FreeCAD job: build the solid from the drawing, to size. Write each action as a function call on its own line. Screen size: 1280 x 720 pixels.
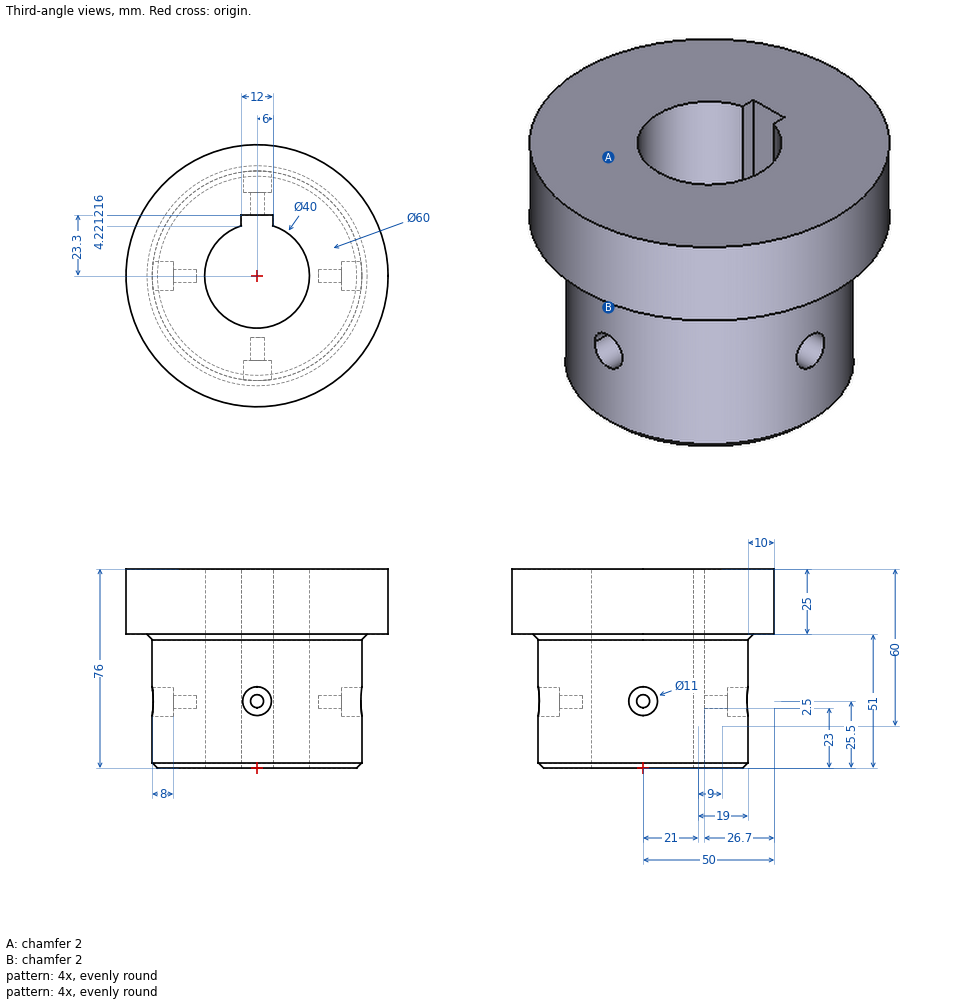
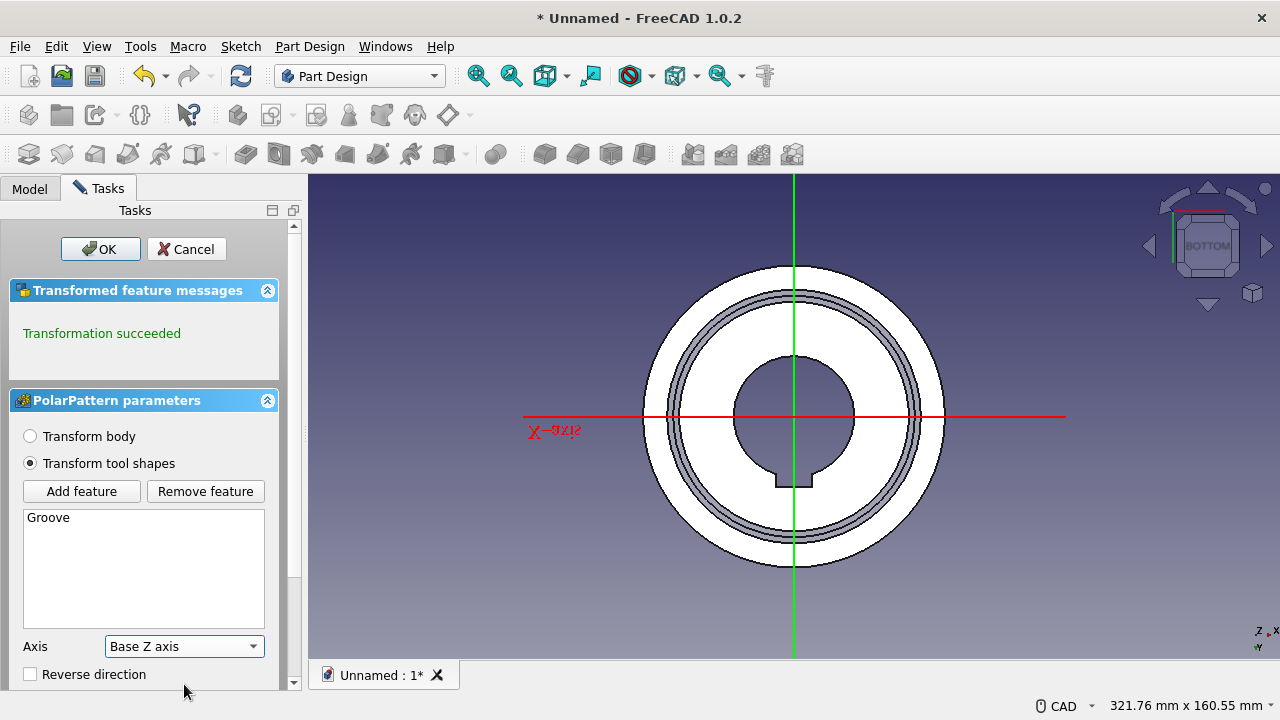
scroll(294, 455, down, 3)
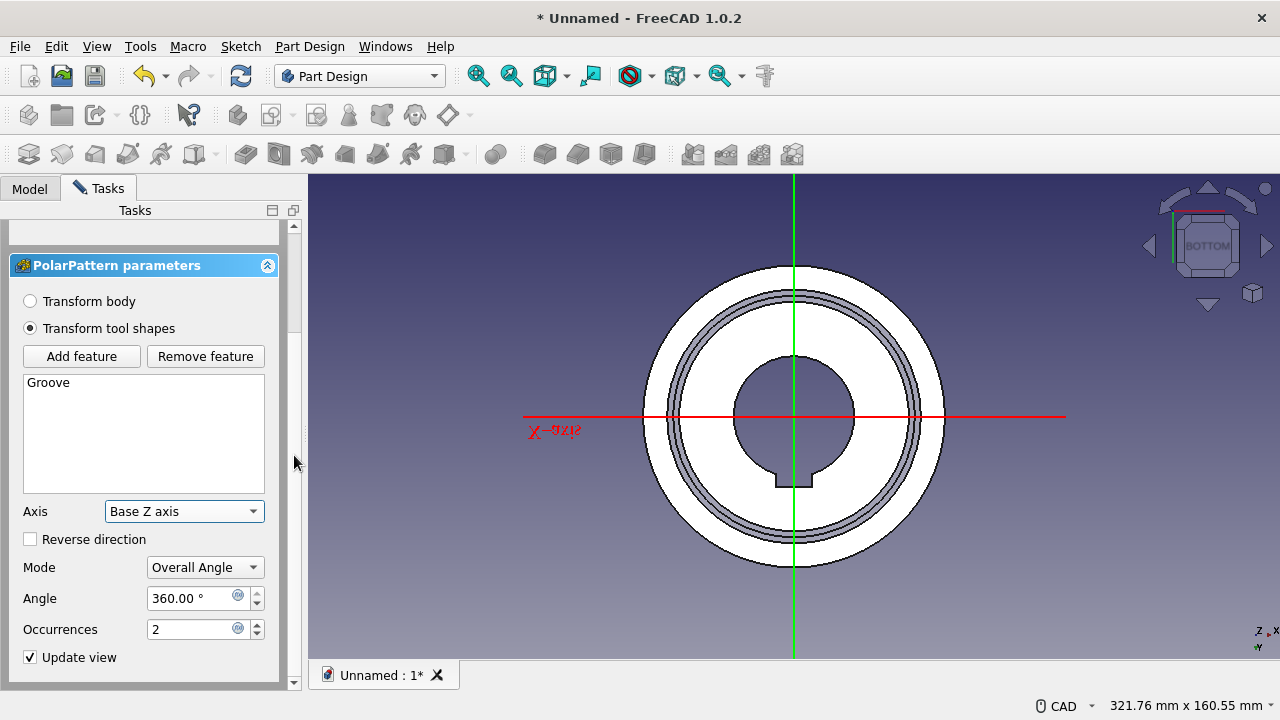
triple_click(199, 630)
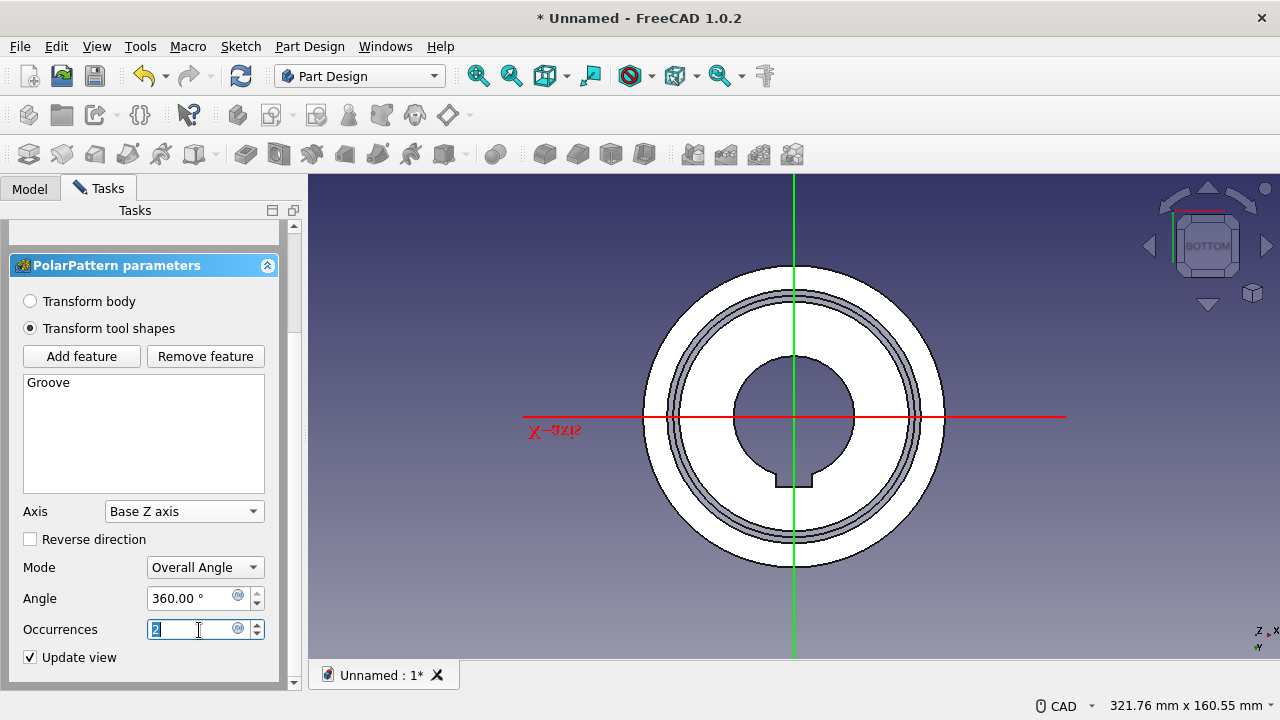
text(4)
key(Tab)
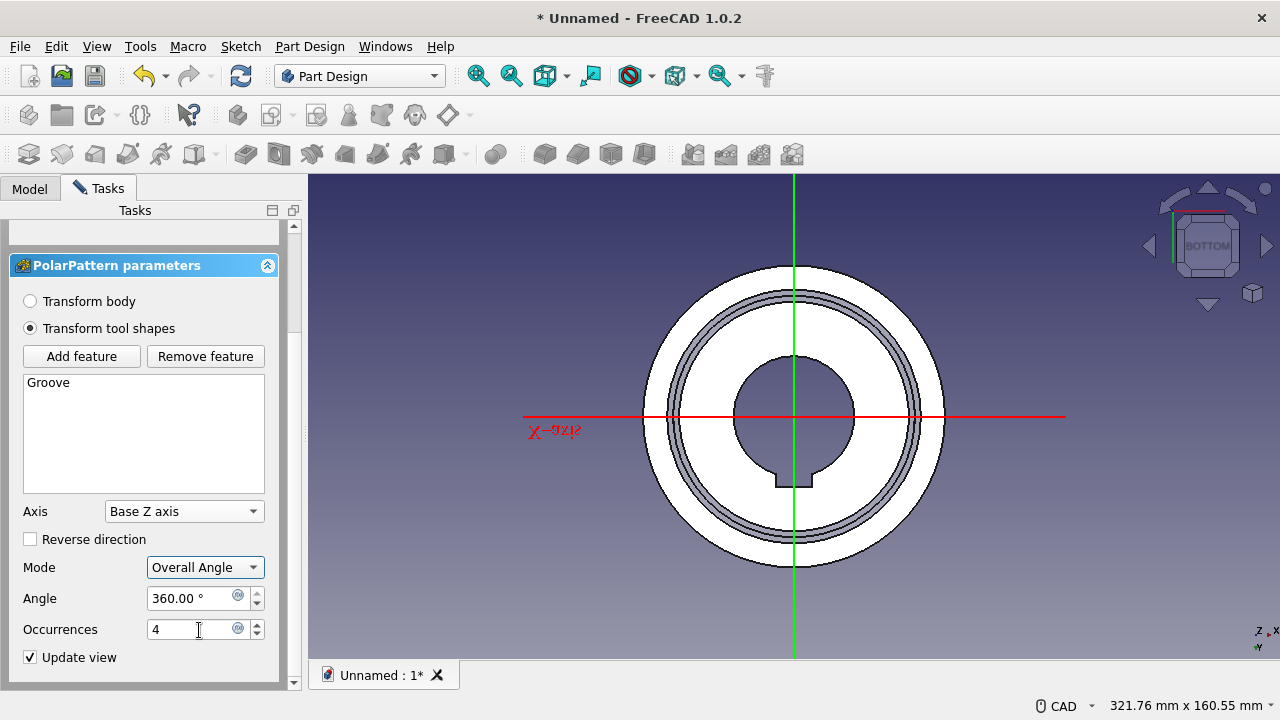
scroll(294, 455, up, 3)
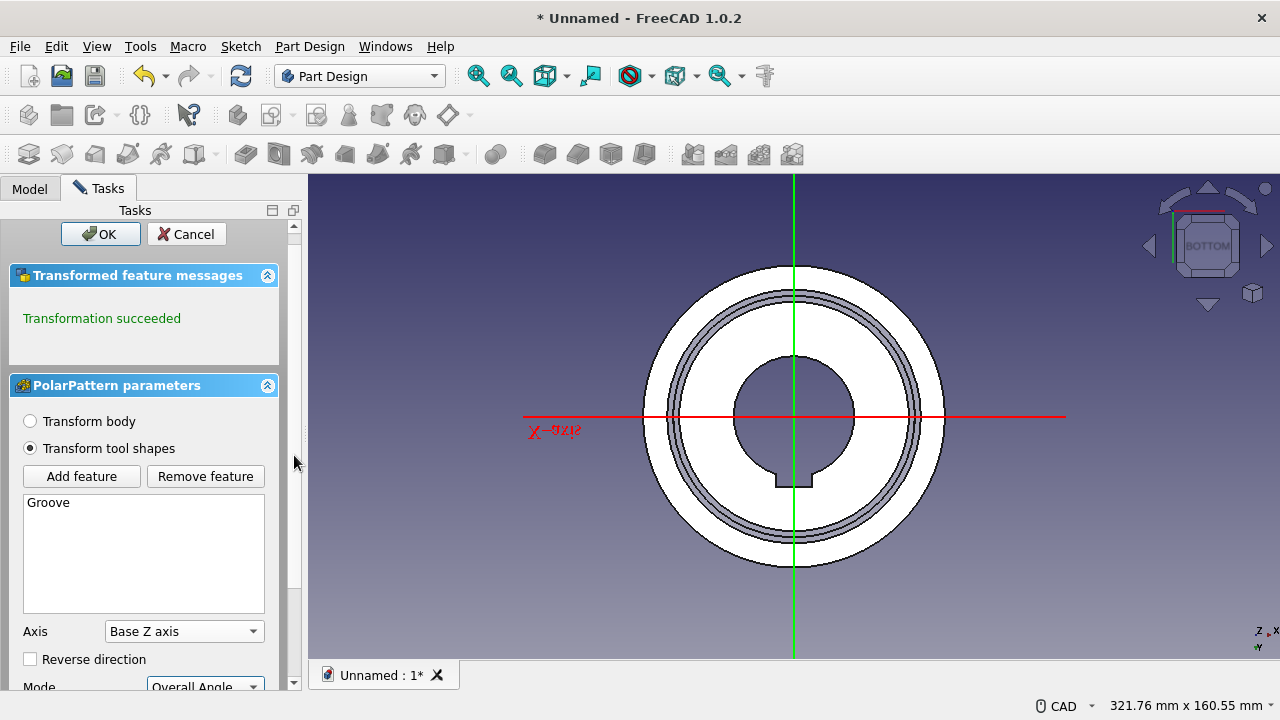
click(101, 249)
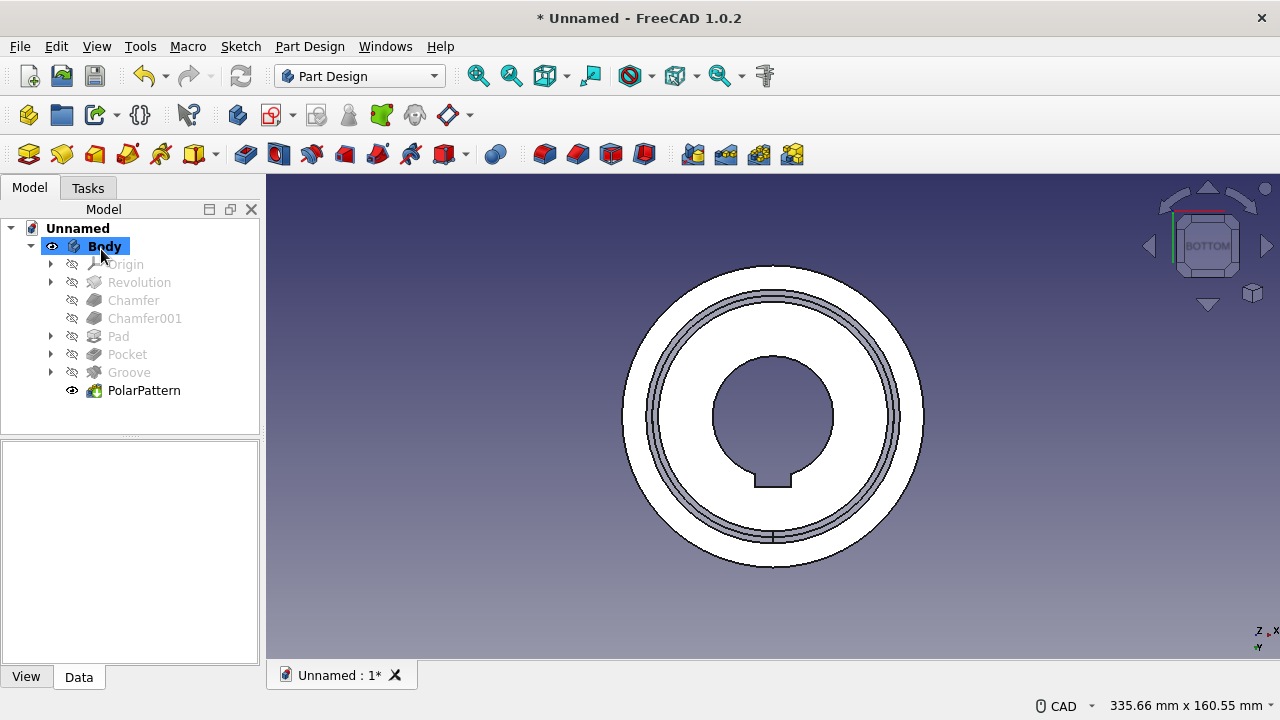
click(51, 264)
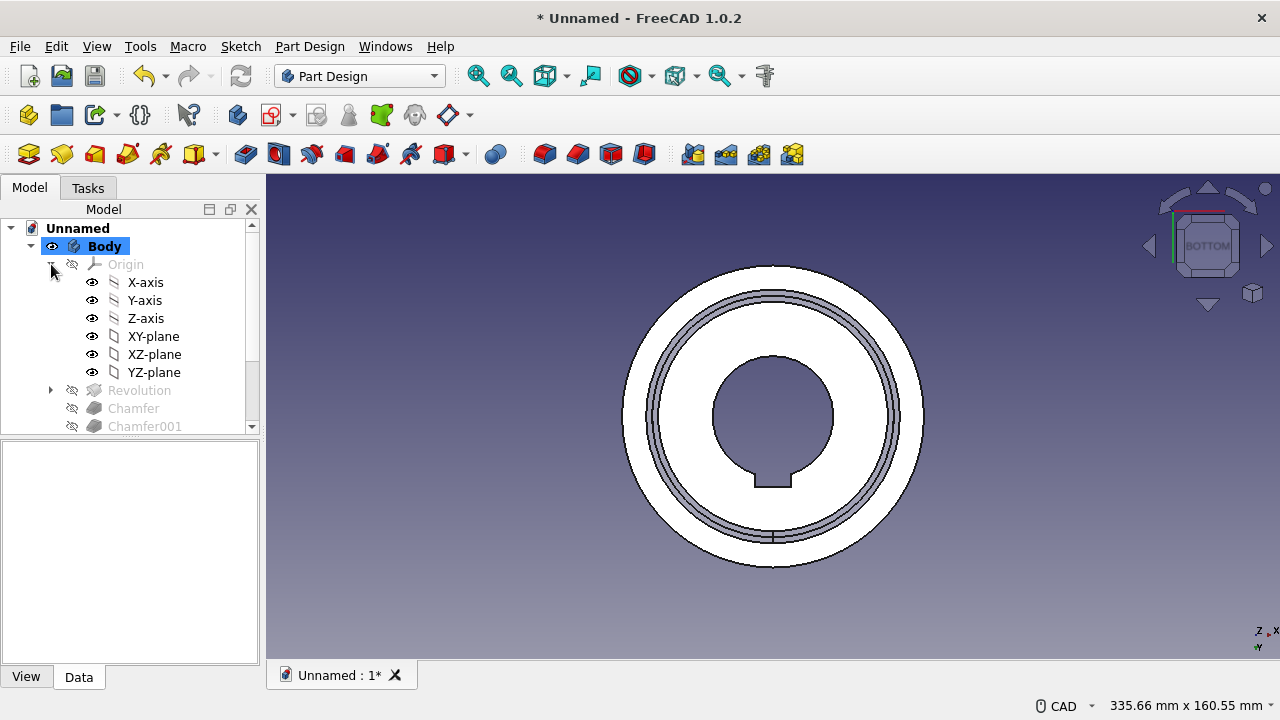
click(137, 372)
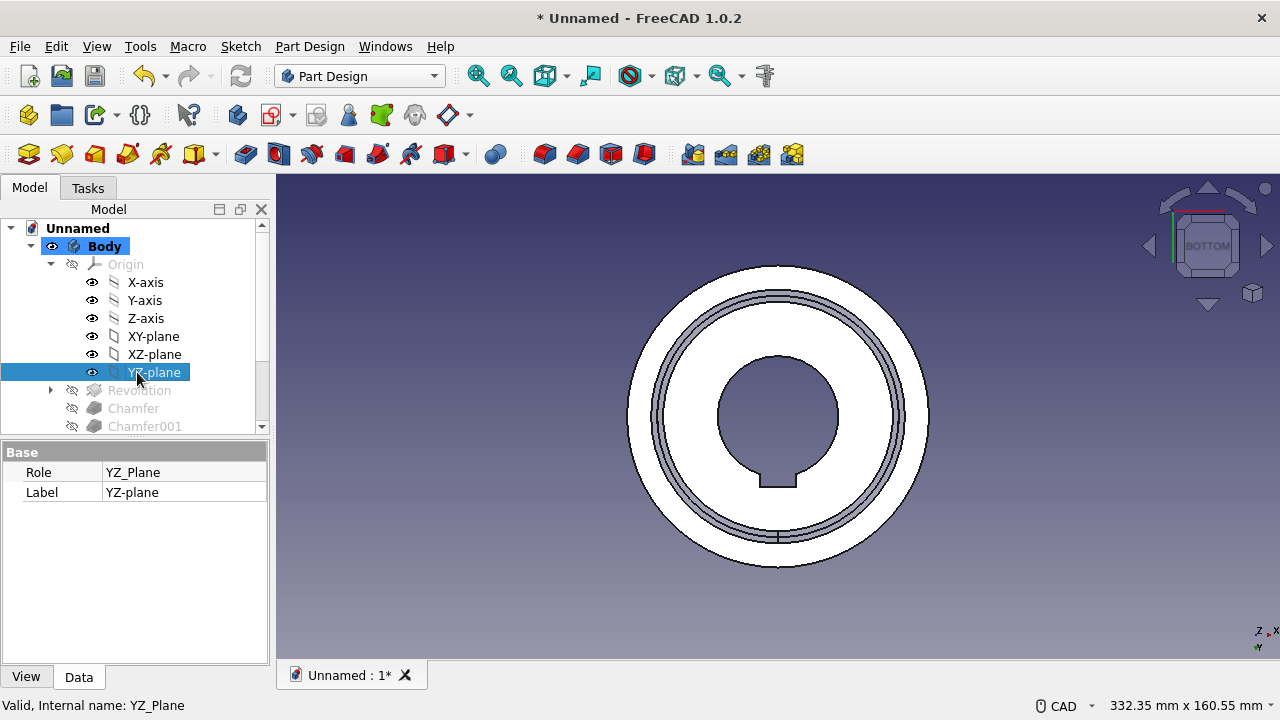
click(448, 116)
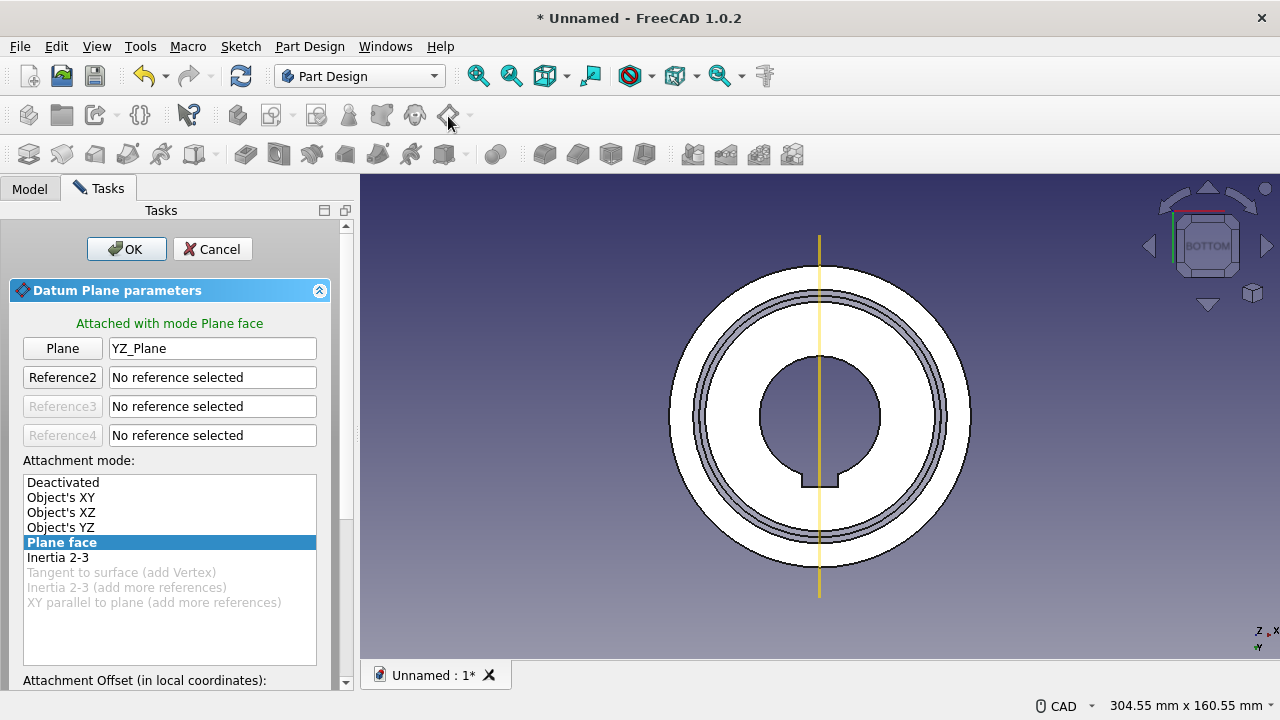
scroll(346, 455, down, 3)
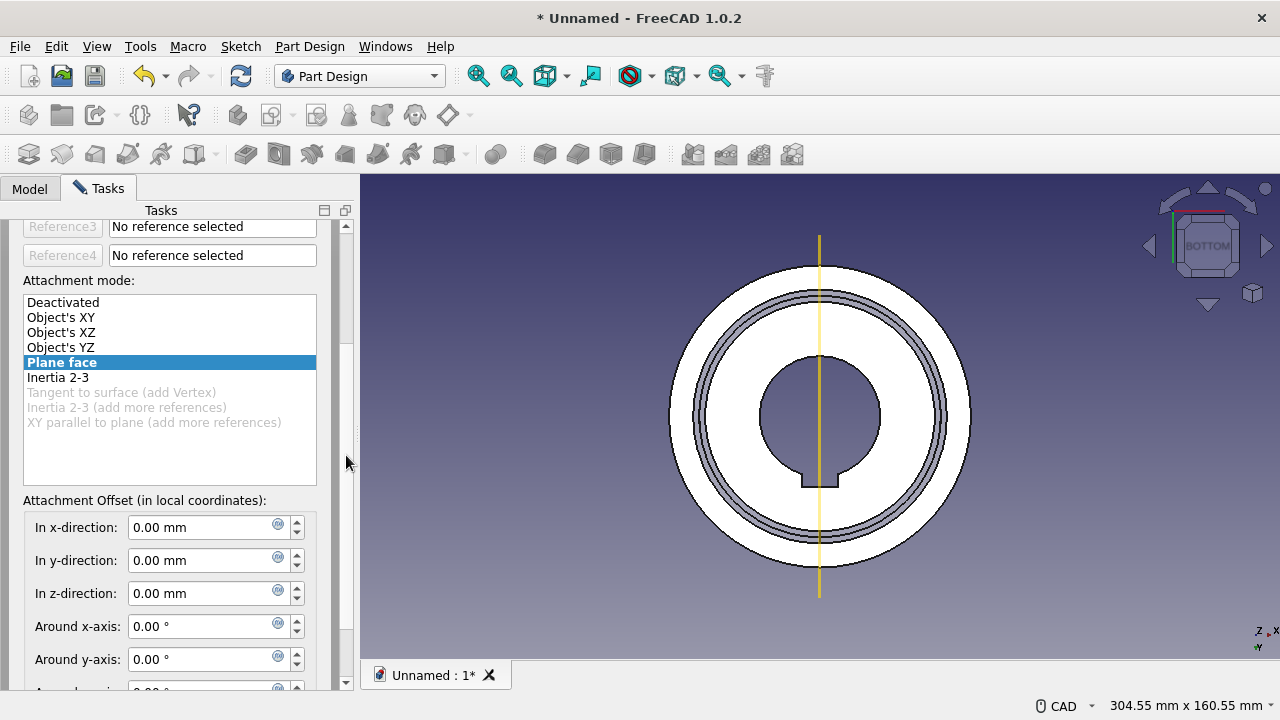
triple_click(210, 594)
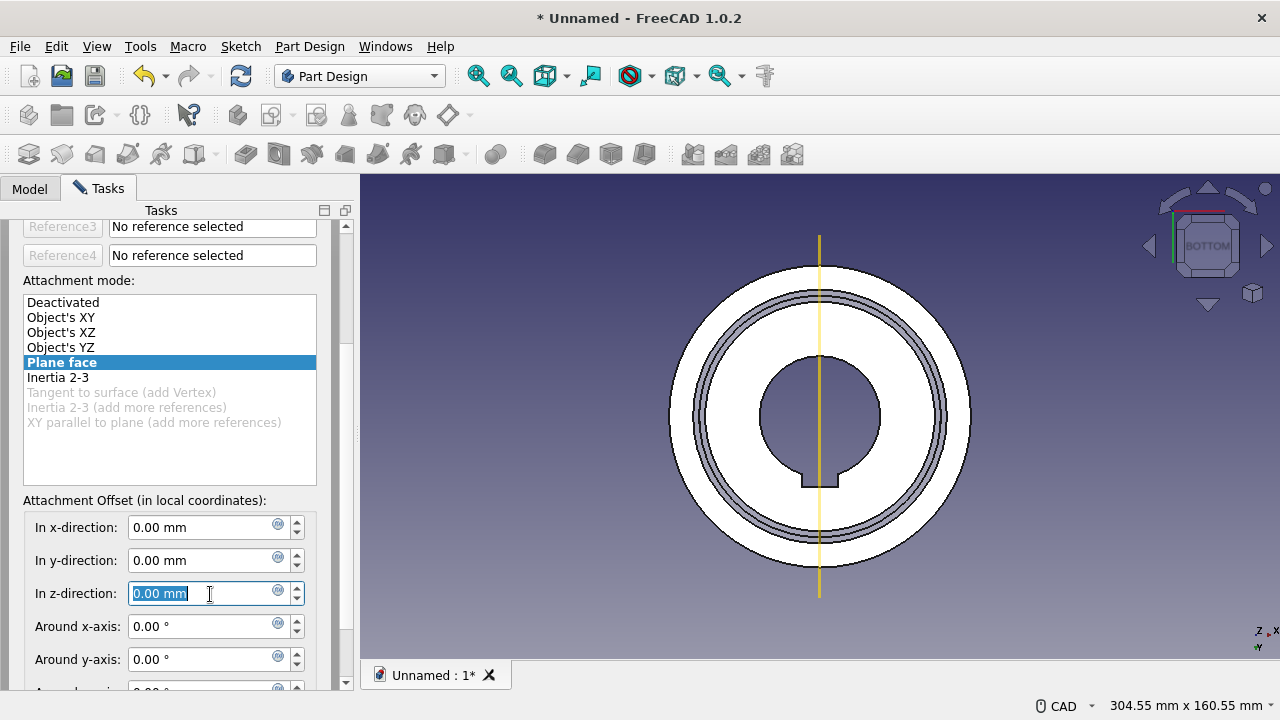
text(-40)
key(Tab)